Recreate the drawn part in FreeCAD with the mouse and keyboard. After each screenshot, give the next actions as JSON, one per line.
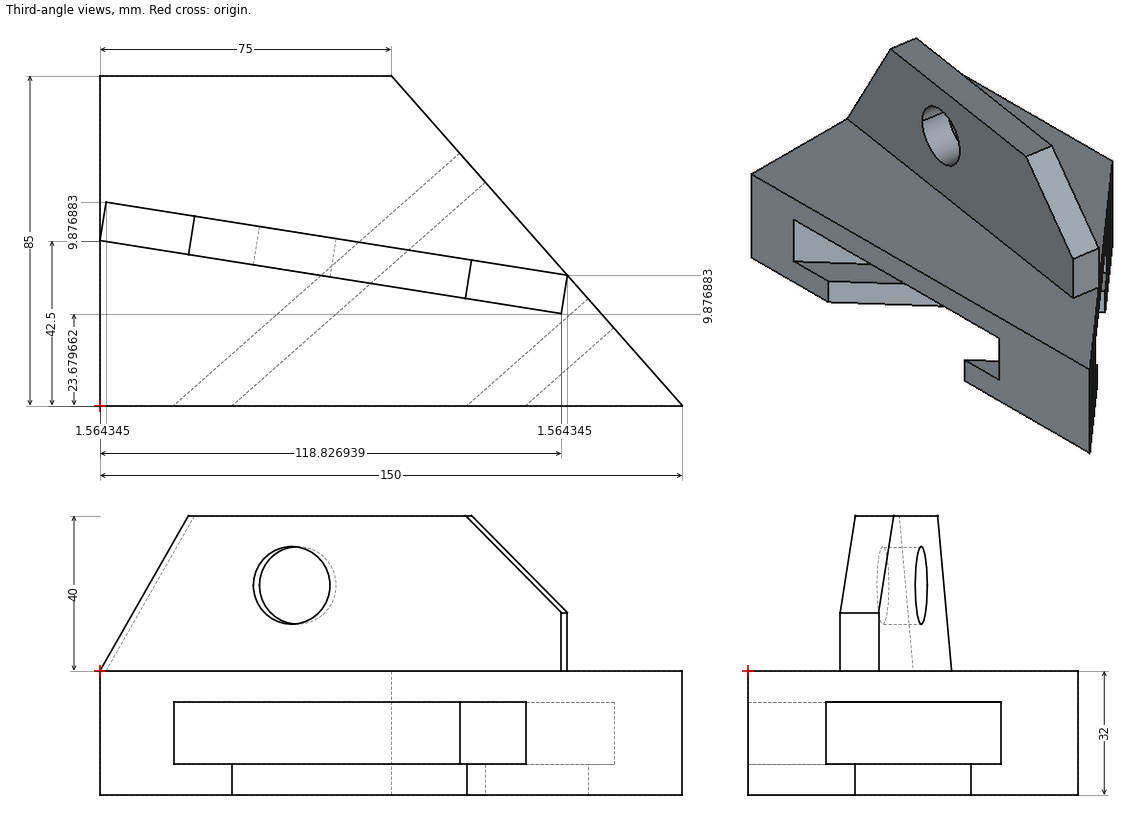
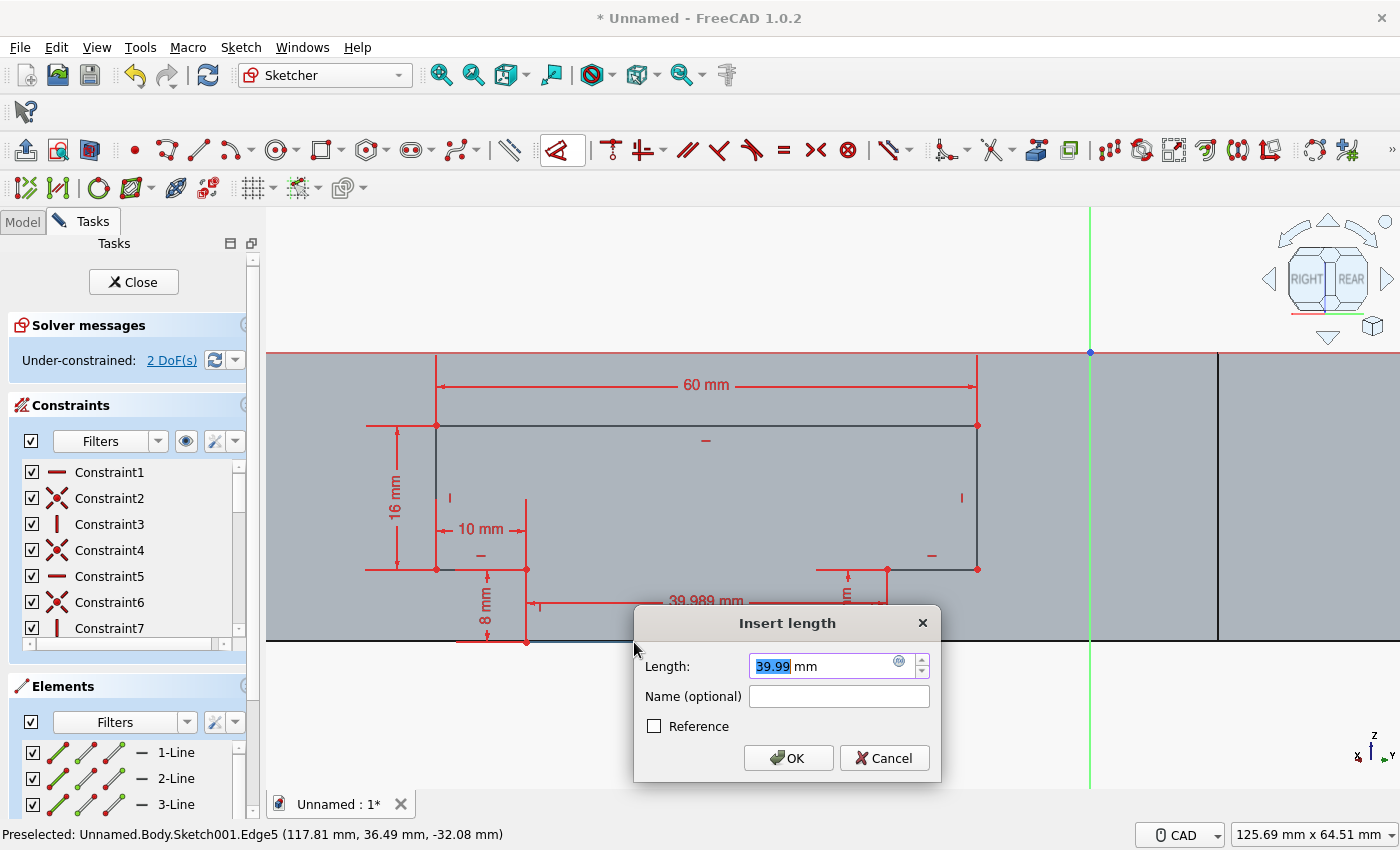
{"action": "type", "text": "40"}
{"action": "key", "text": "Return"}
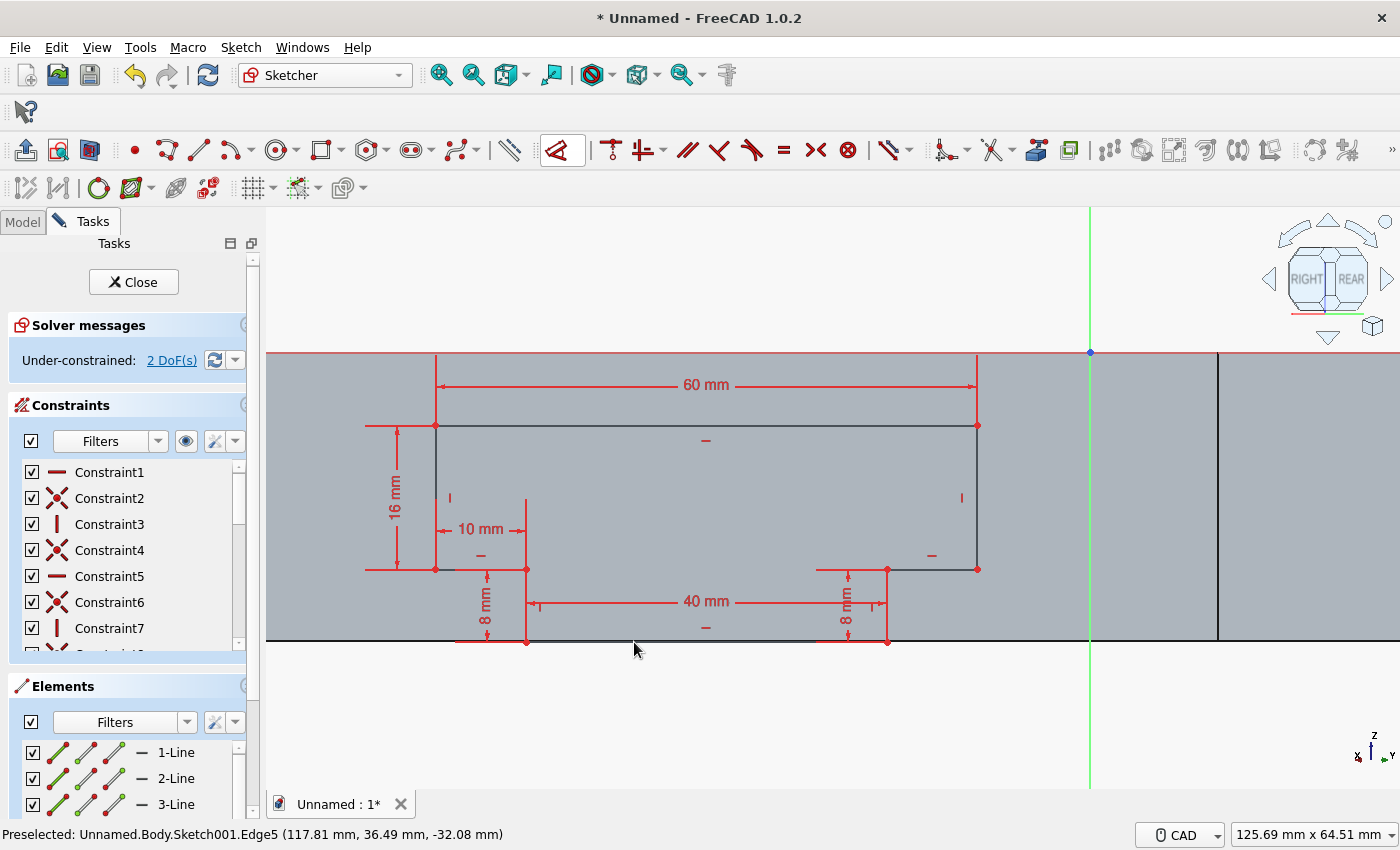
{"action": "left_click", "coordinate": [977, 426]}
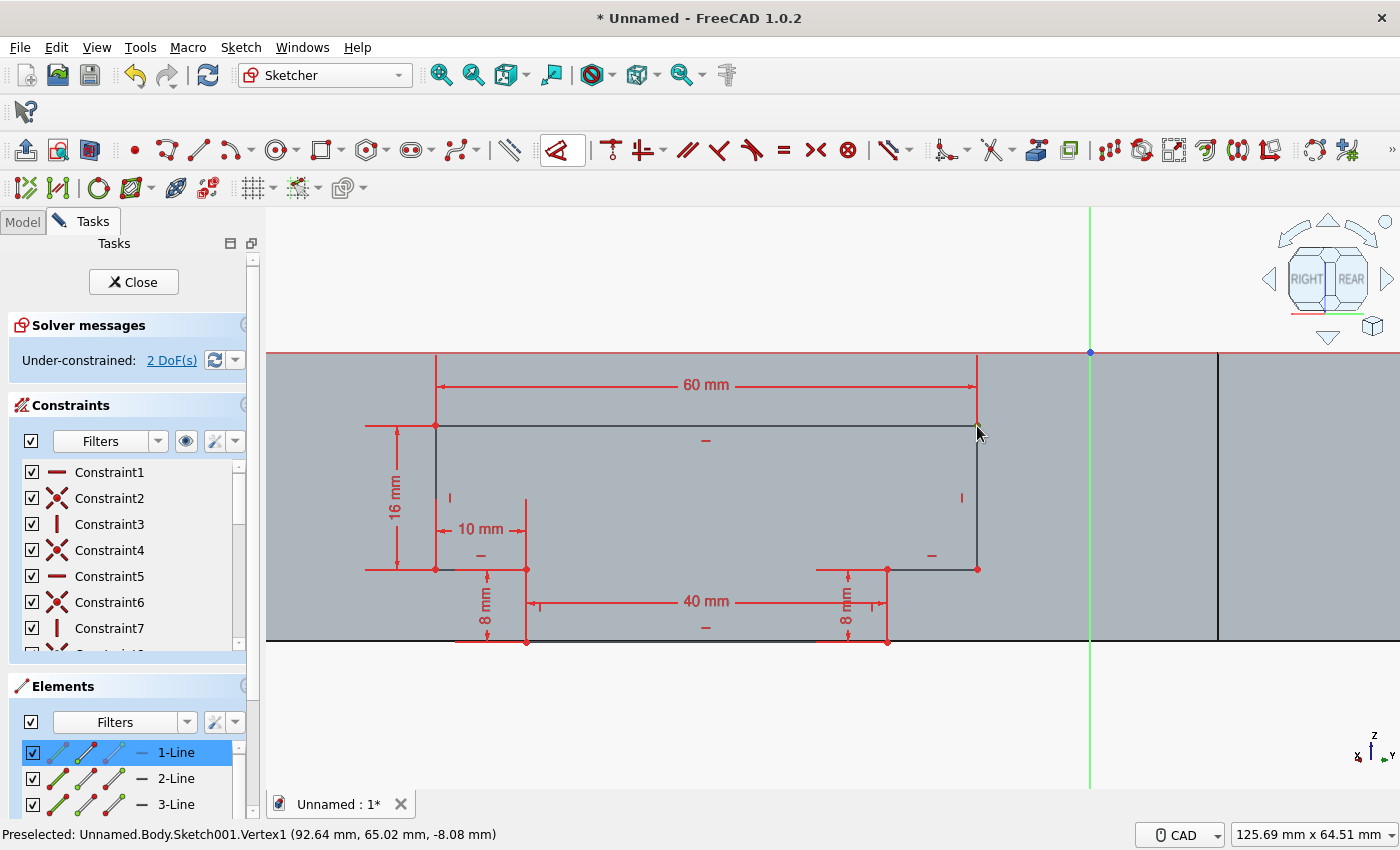
{"action": "key", "text": "i"}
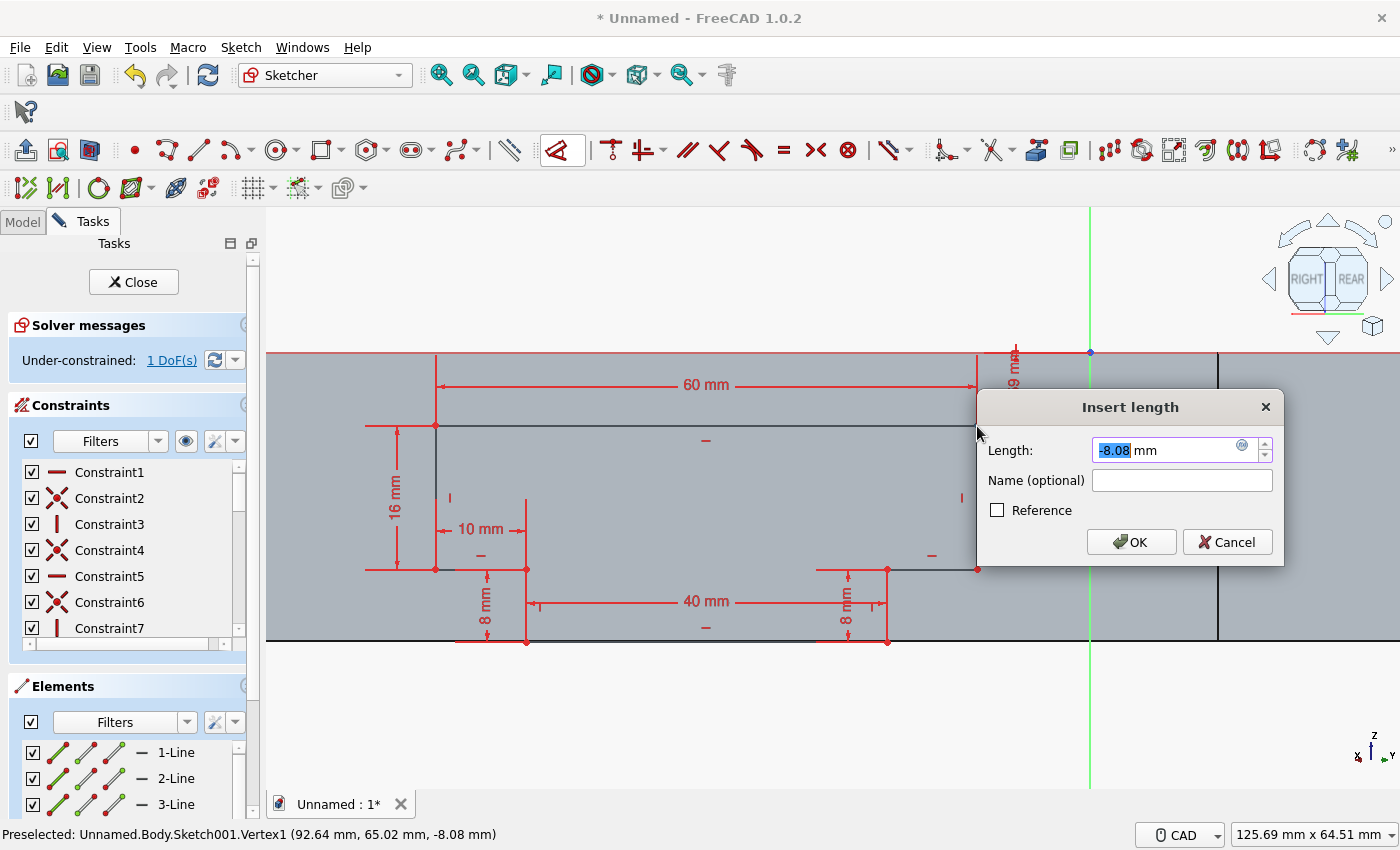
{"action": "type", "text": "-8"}
{"action": "key", "text": "Return"}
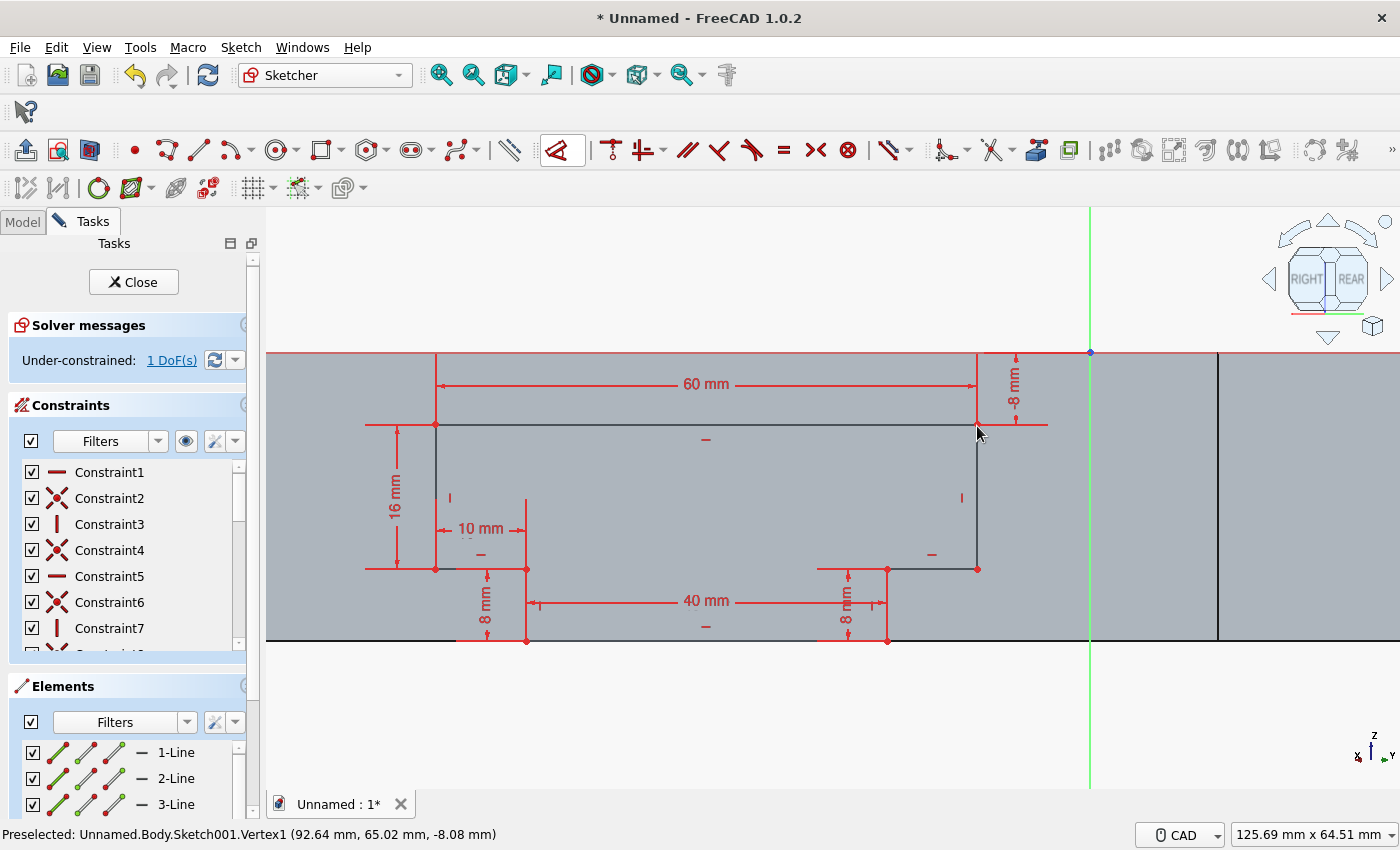
{"action": "left_click", "coordinate": [977, 425]}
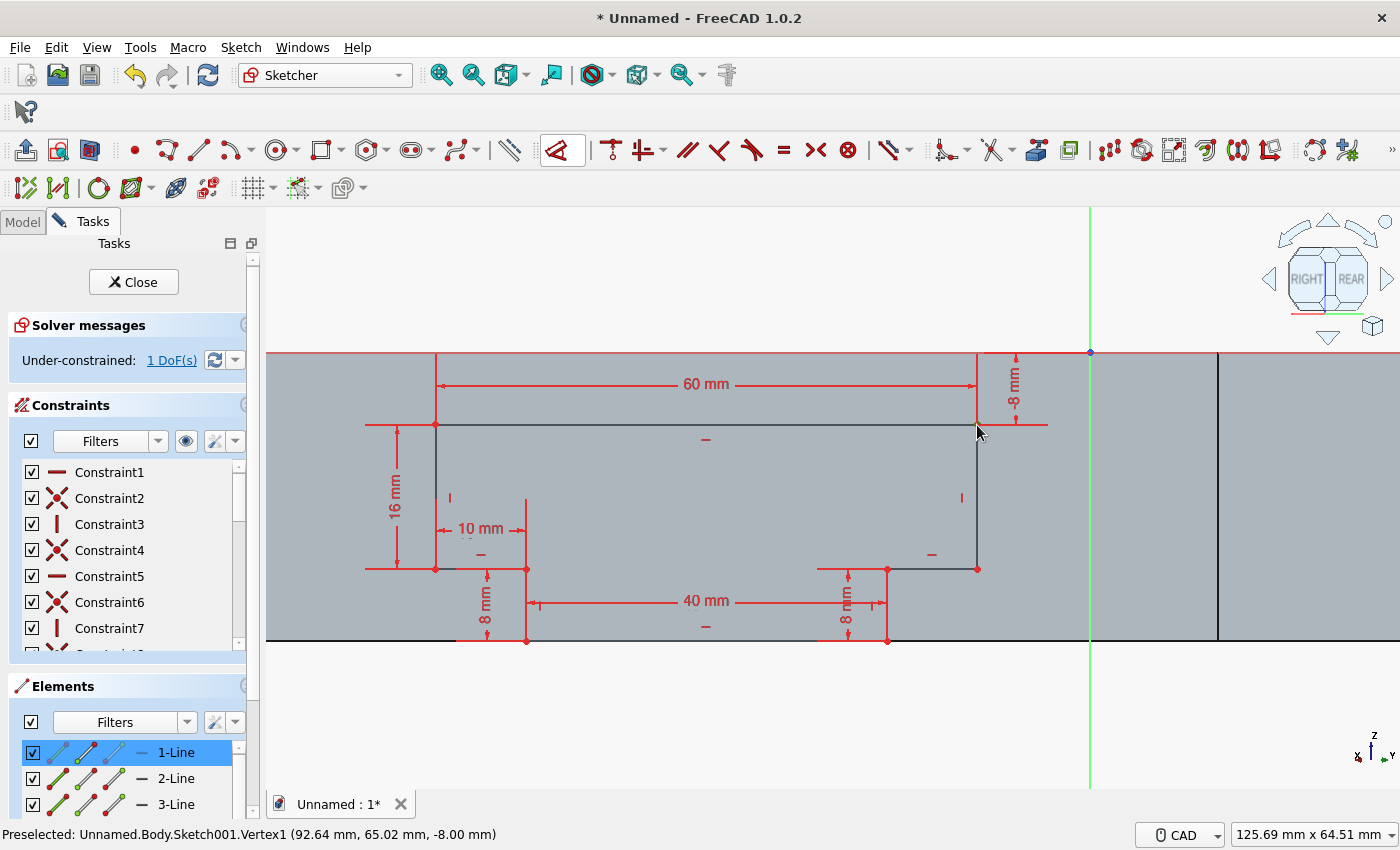
{"action": "key", "text": "l"}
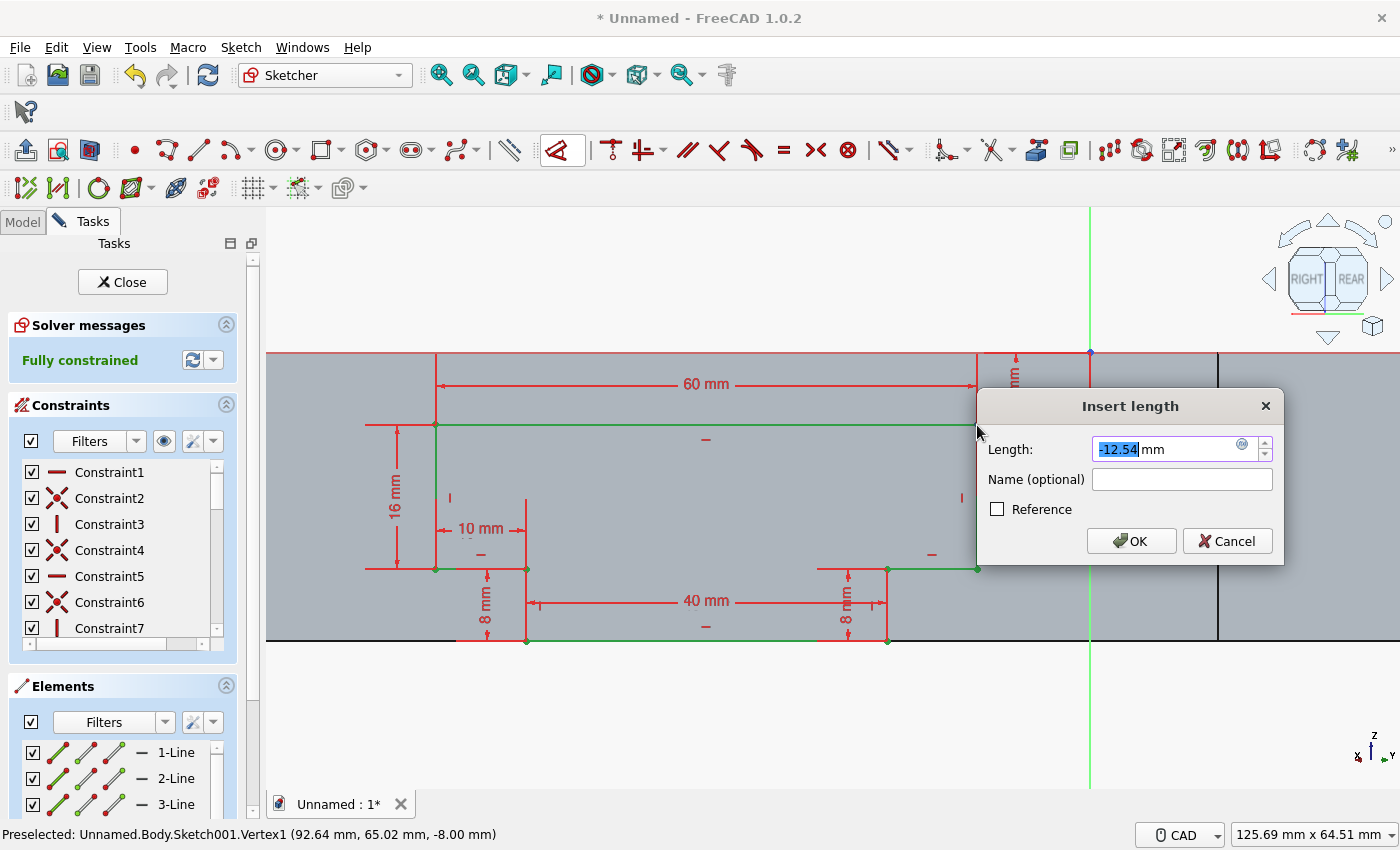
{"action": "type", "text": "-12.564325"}
{"action": "key", "text": "Return"}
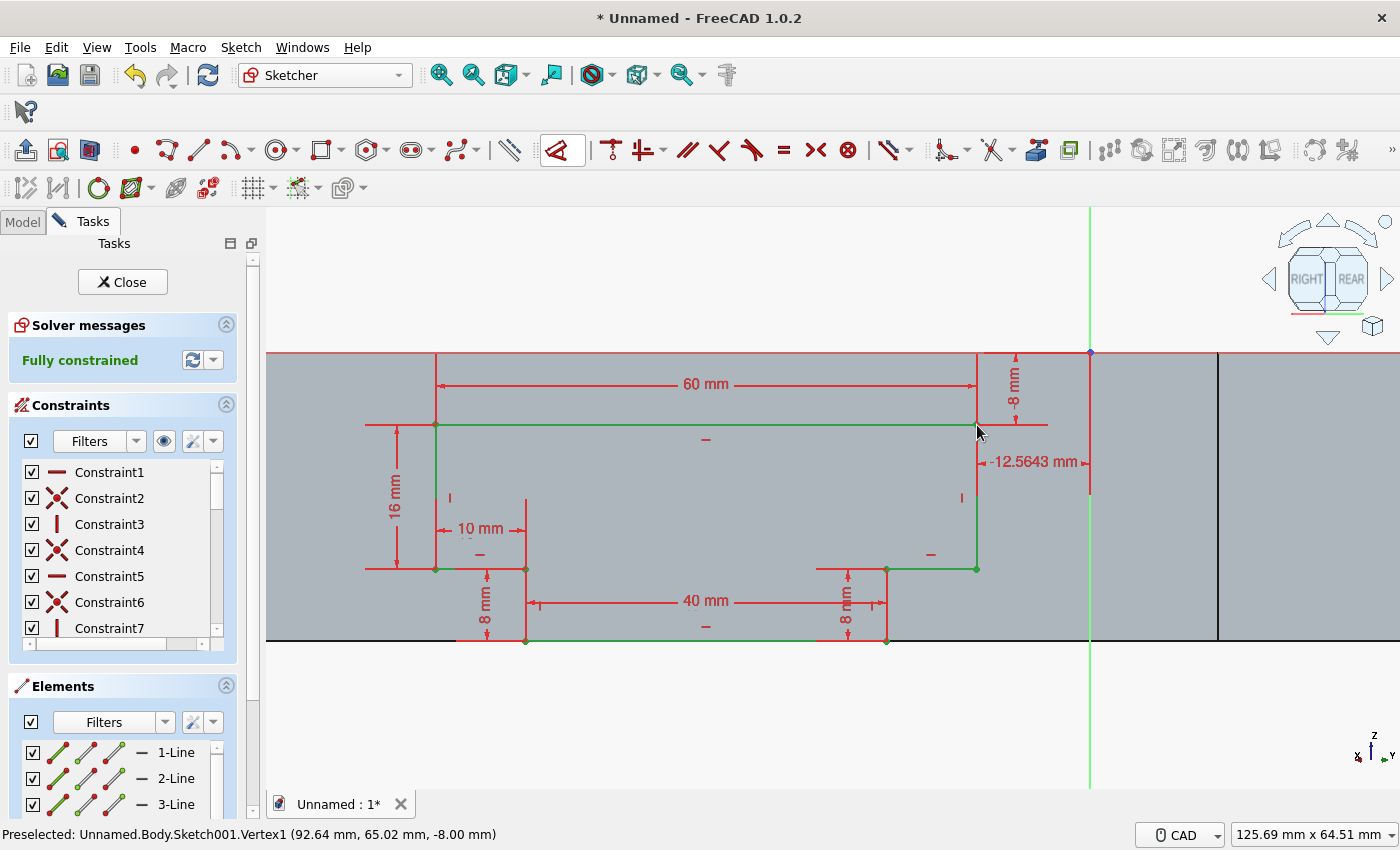
{"action": "left_click", "coordinate": [123, 282]}